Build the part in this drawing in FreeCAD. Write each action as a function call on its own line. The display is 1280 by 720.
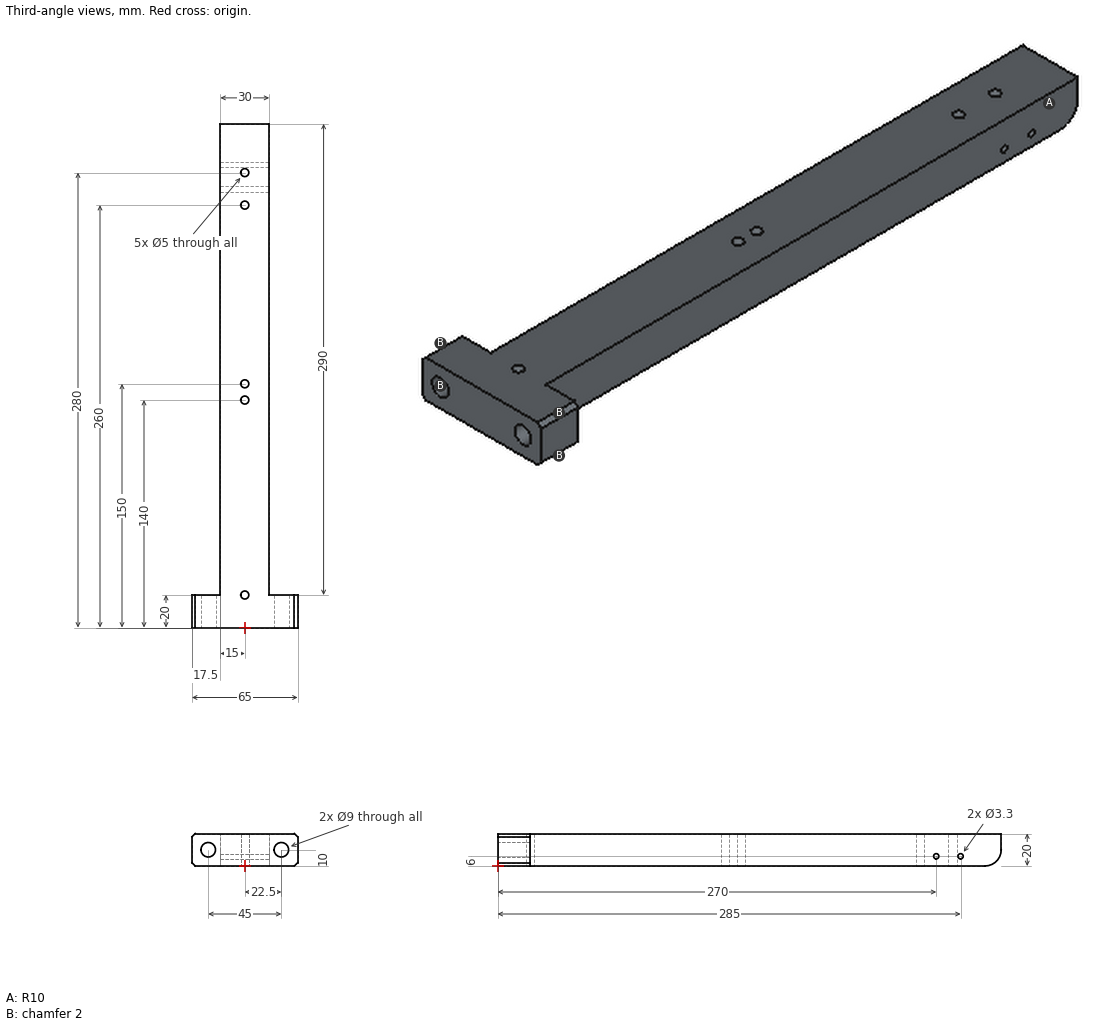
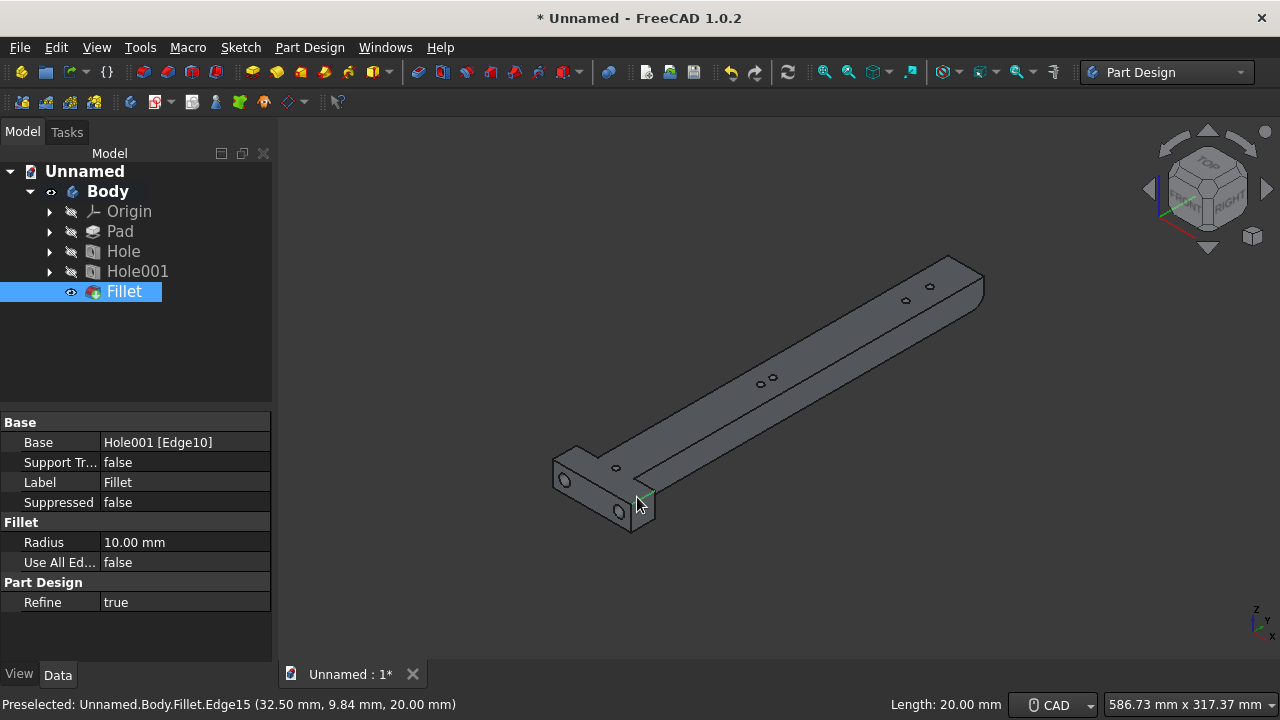
key(2)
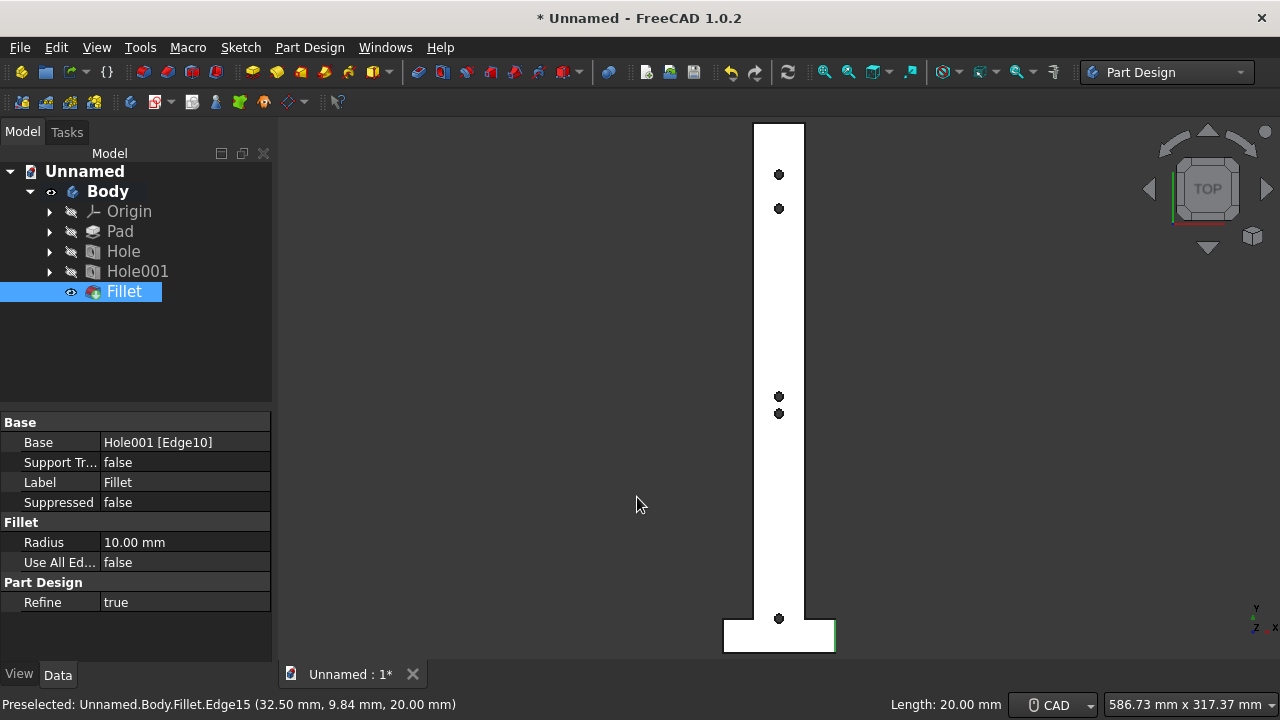
click(723, 628, ctrl)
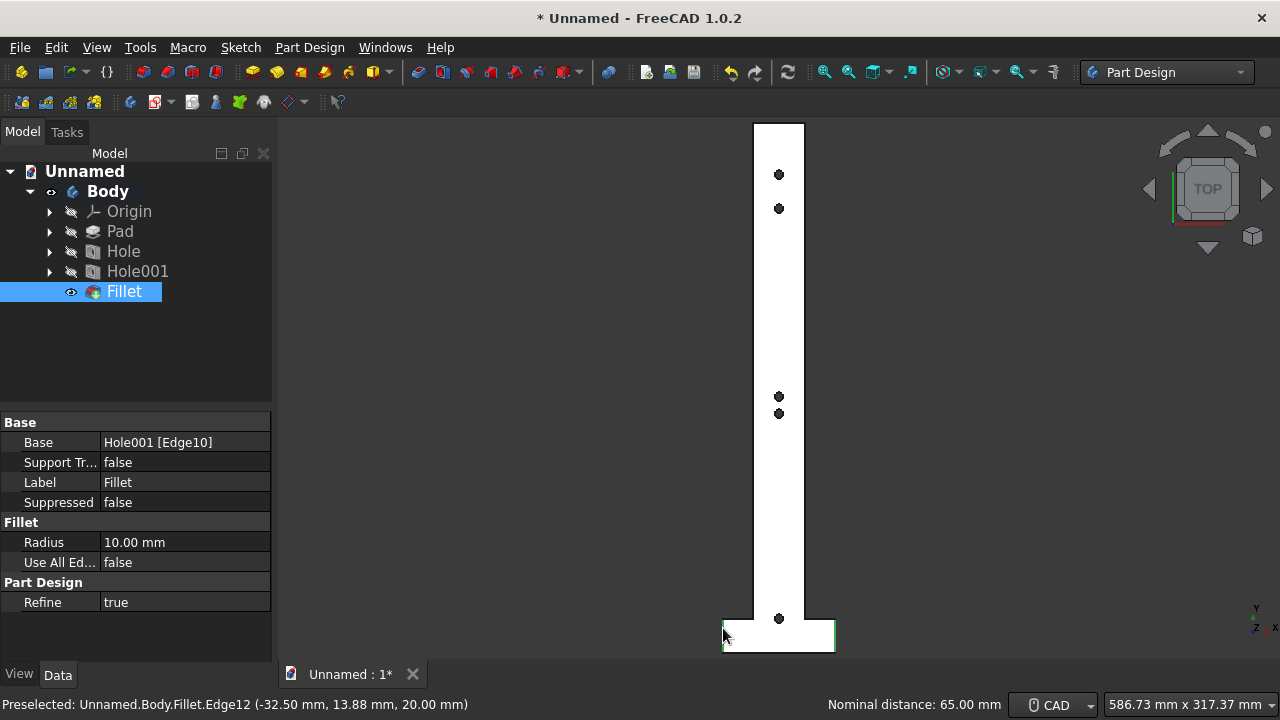
key(1)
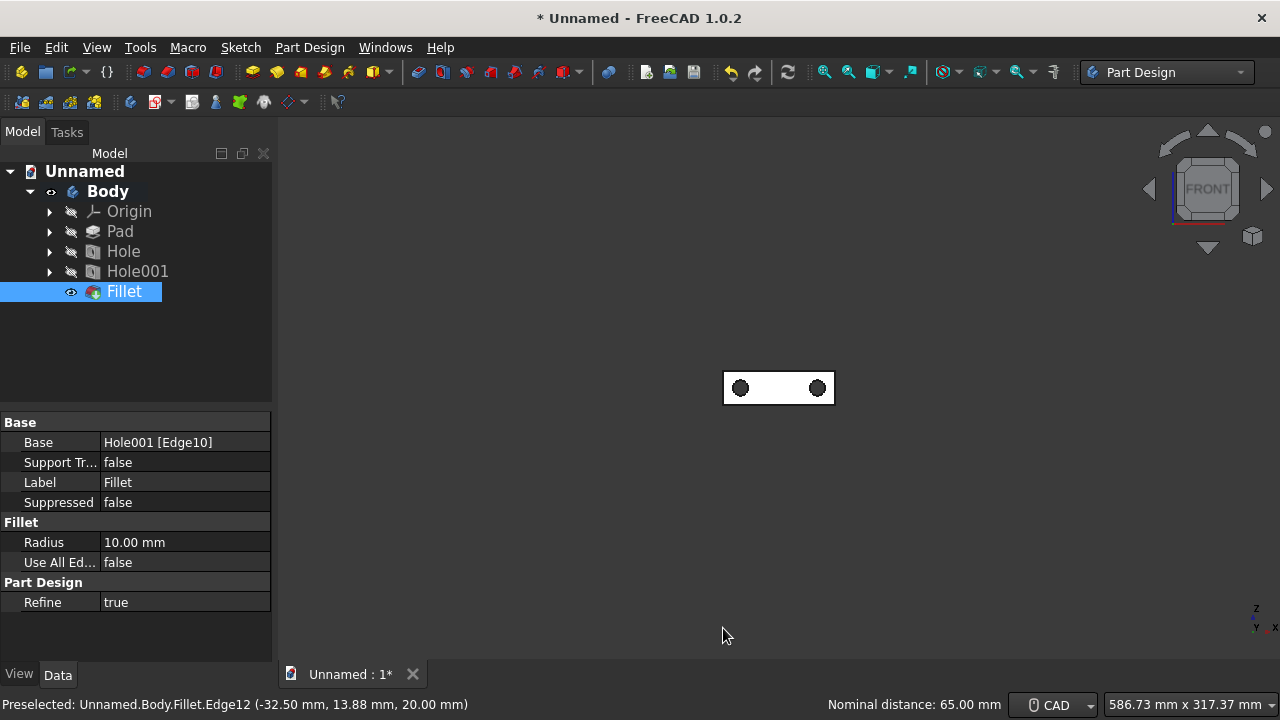
click(826, 72)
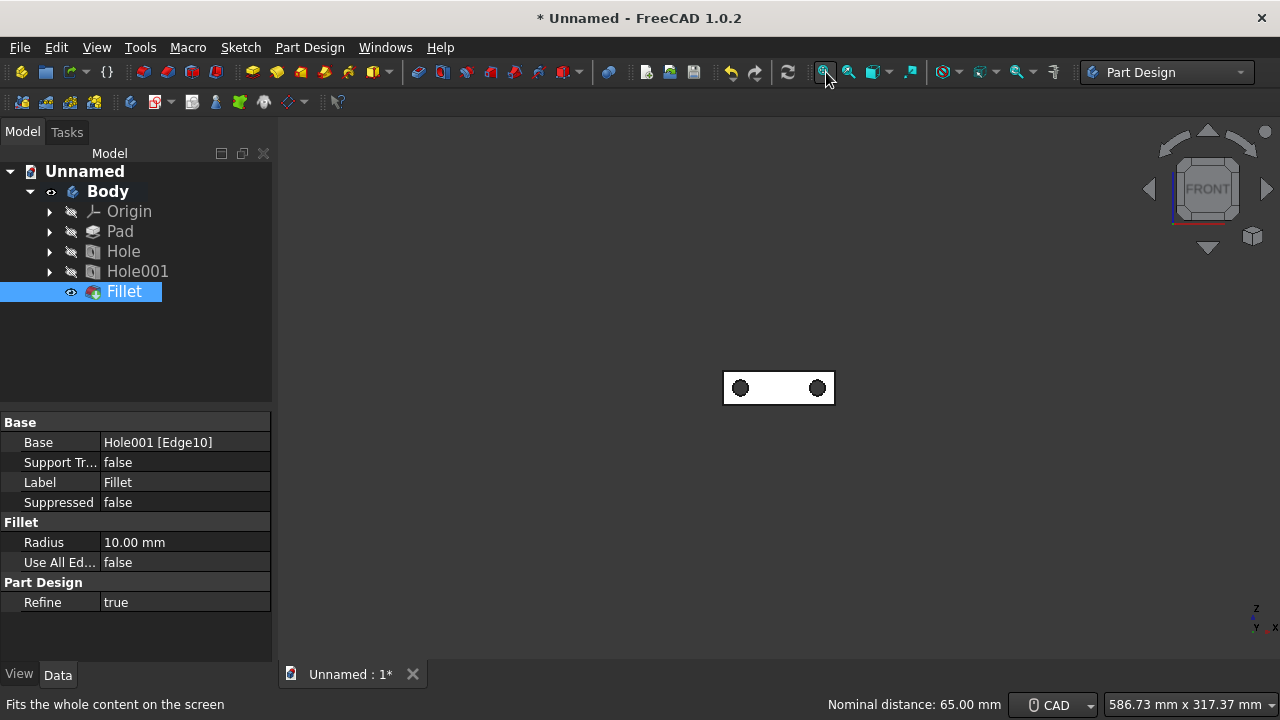
key(3)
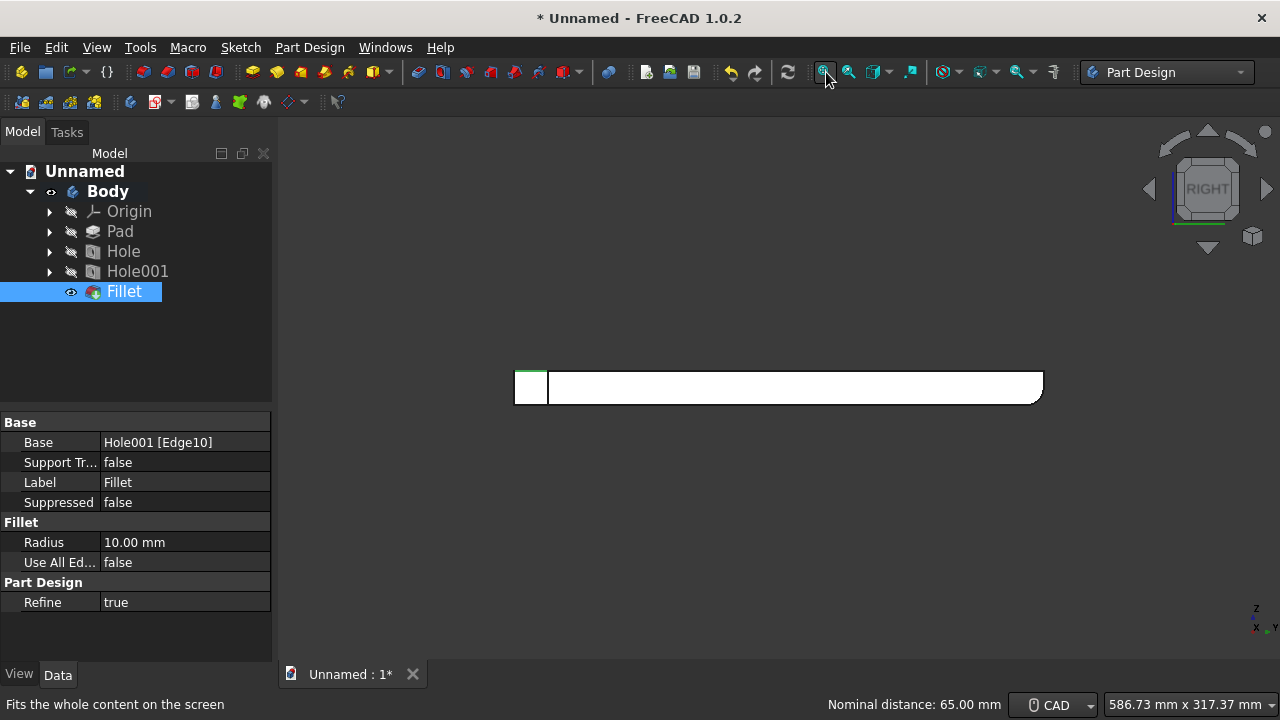
click(531, 404, ctrl)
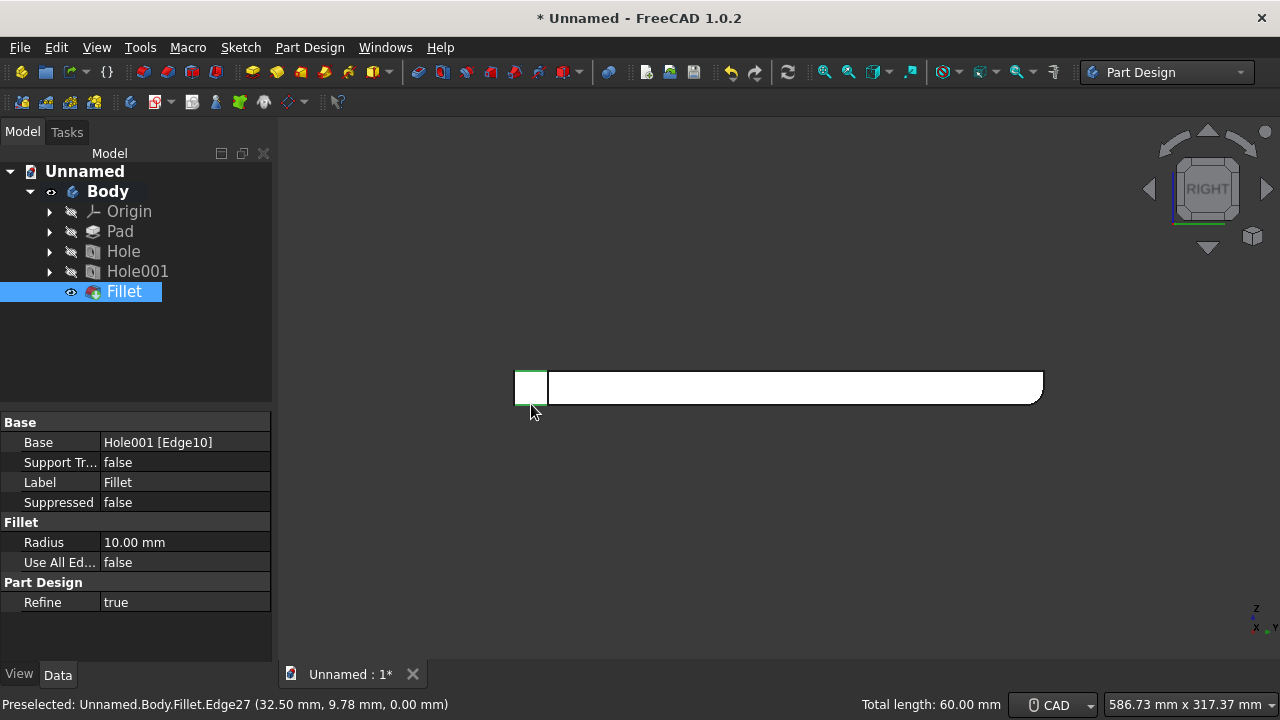
key(5)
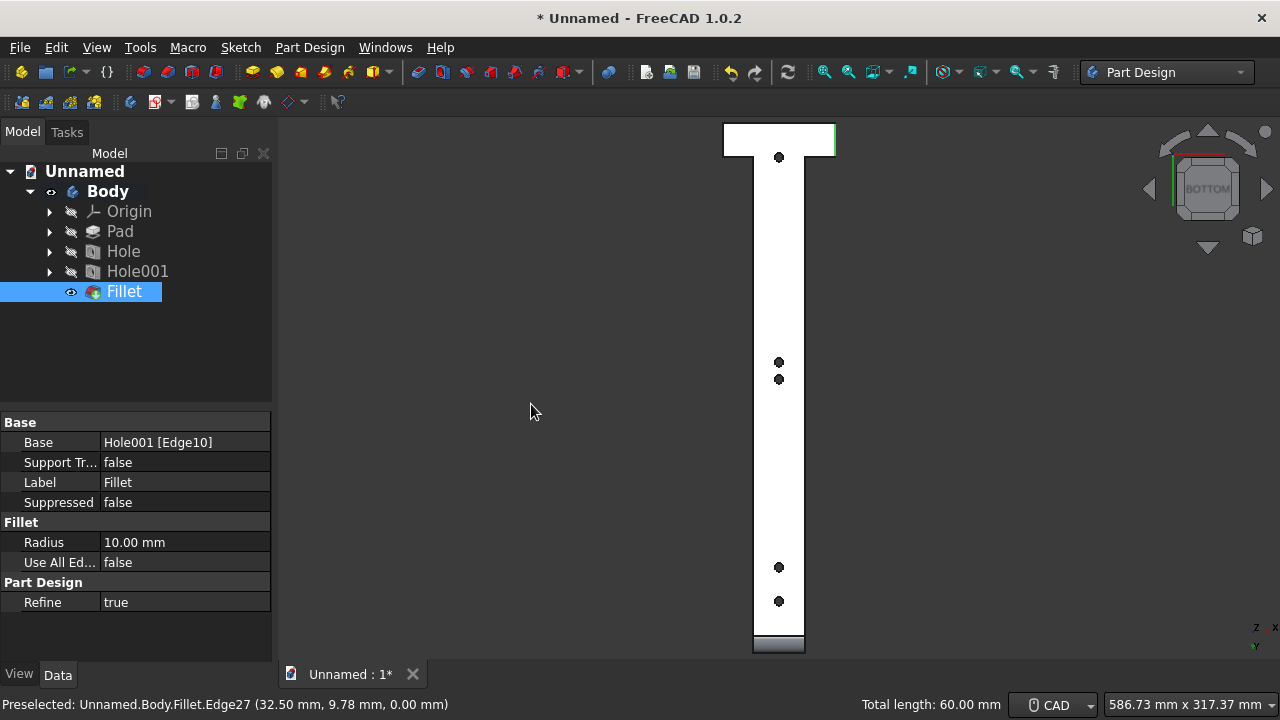
click(723, 146, ctrl)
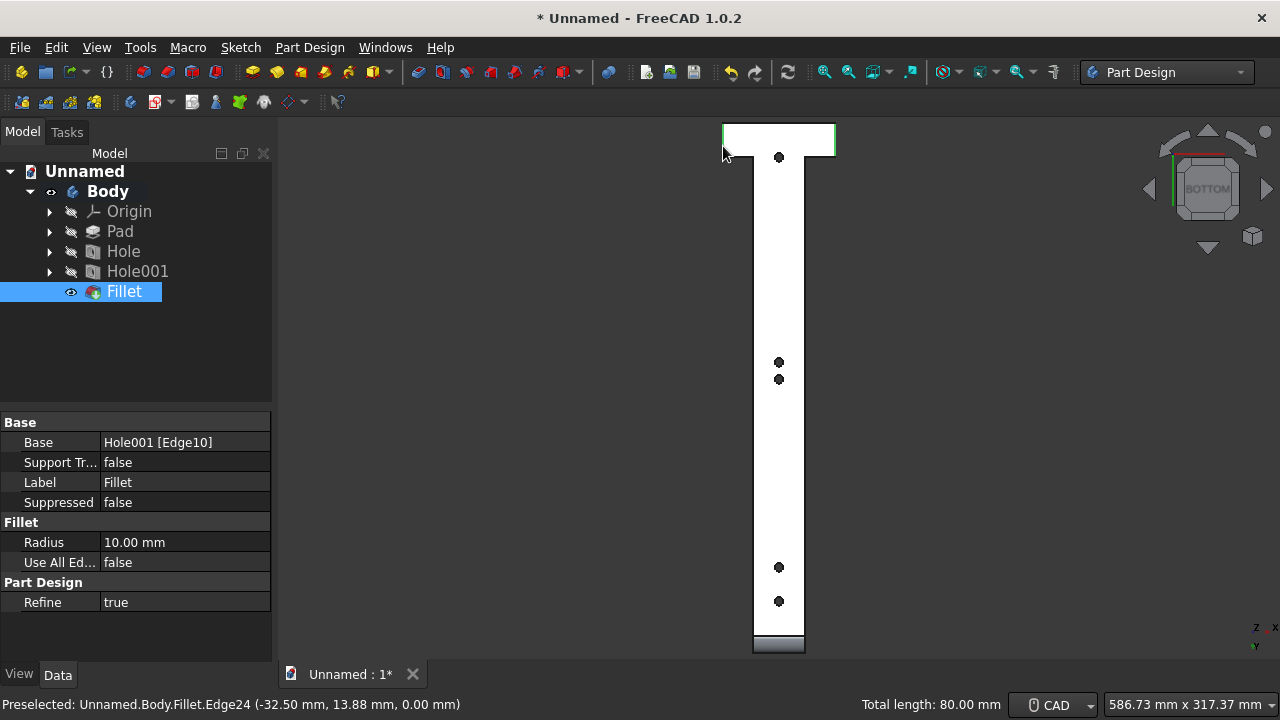
click(168, 72)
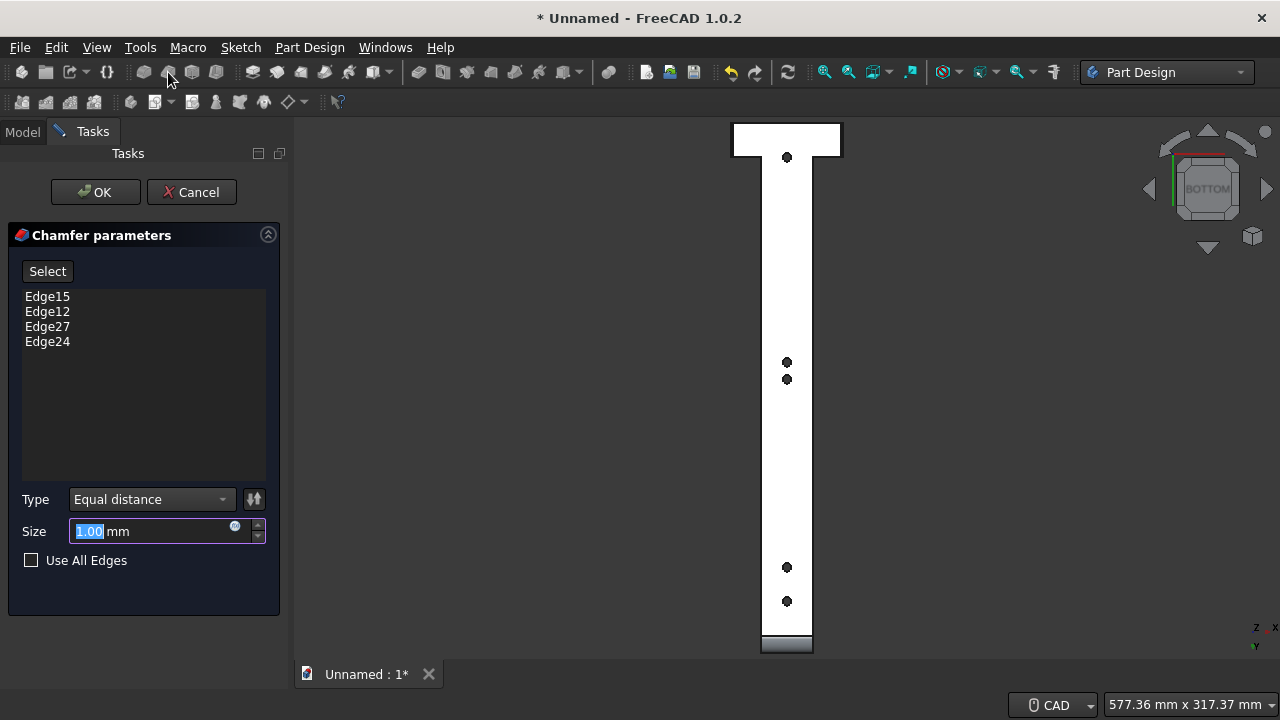
text(2)
key(Tab)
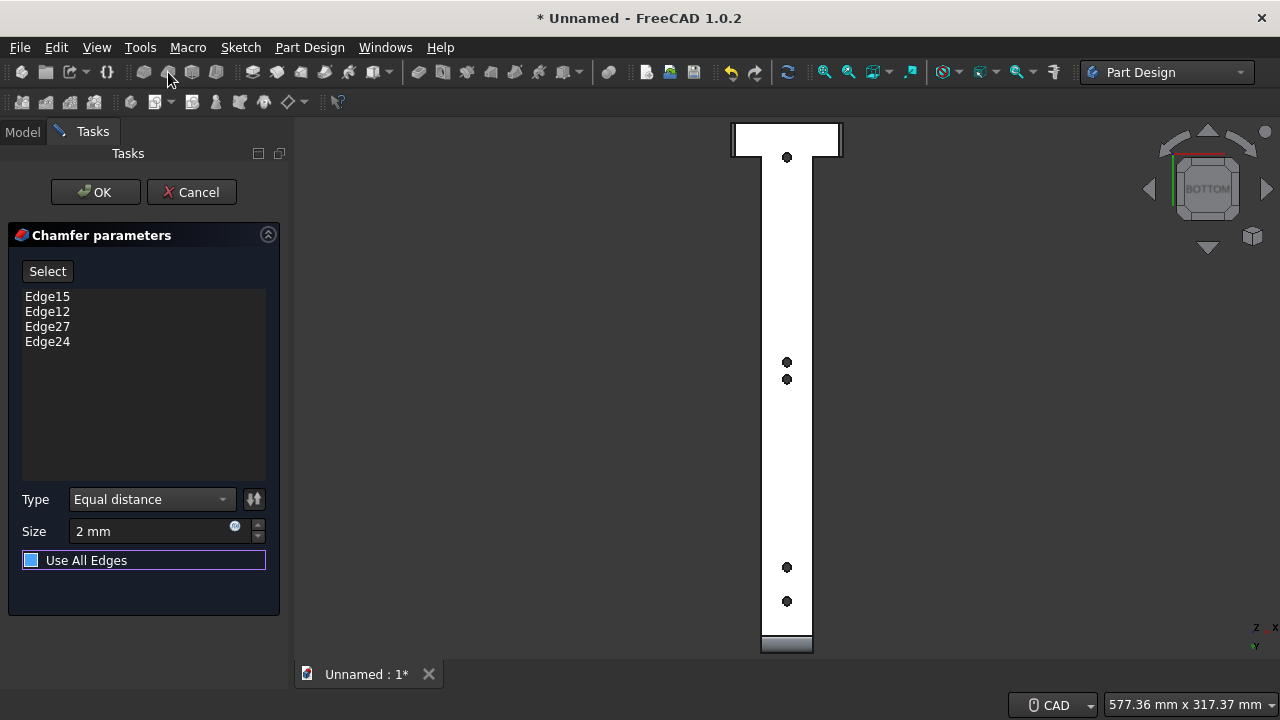
click(96, 192)